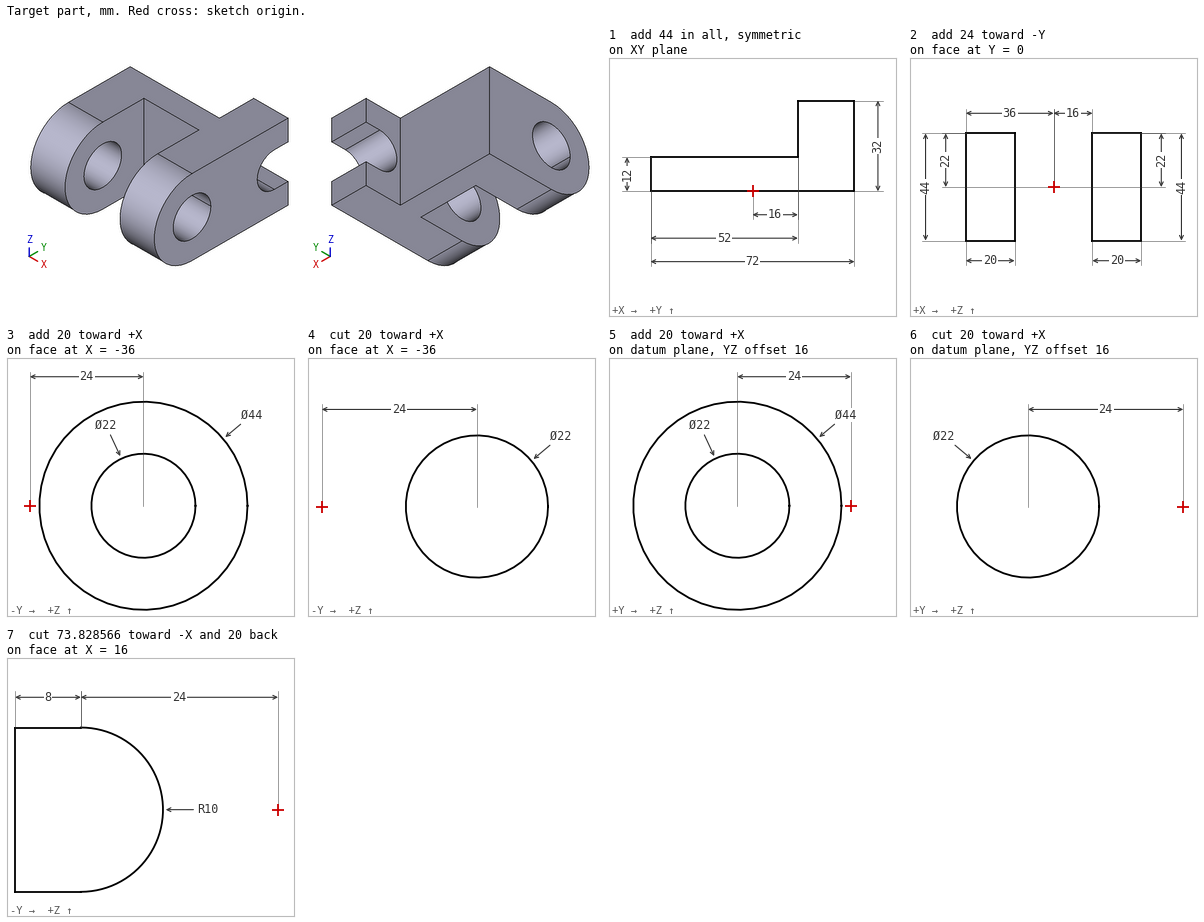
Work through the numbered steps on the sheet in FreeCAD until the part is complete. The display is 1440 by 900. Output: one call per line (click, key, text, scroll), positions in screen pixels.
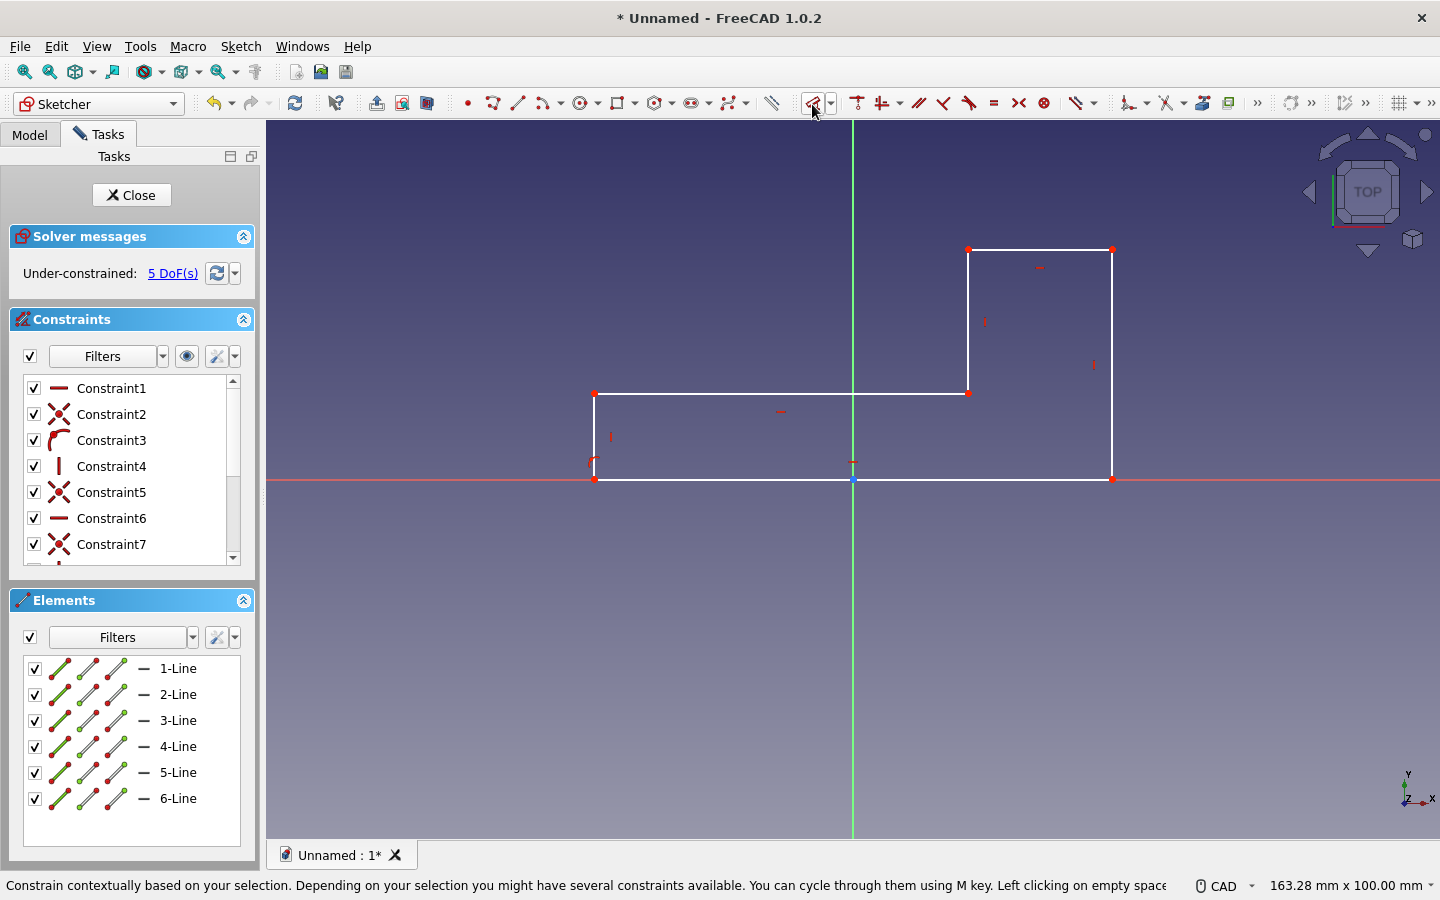
click(856, 394)
click(781, 428)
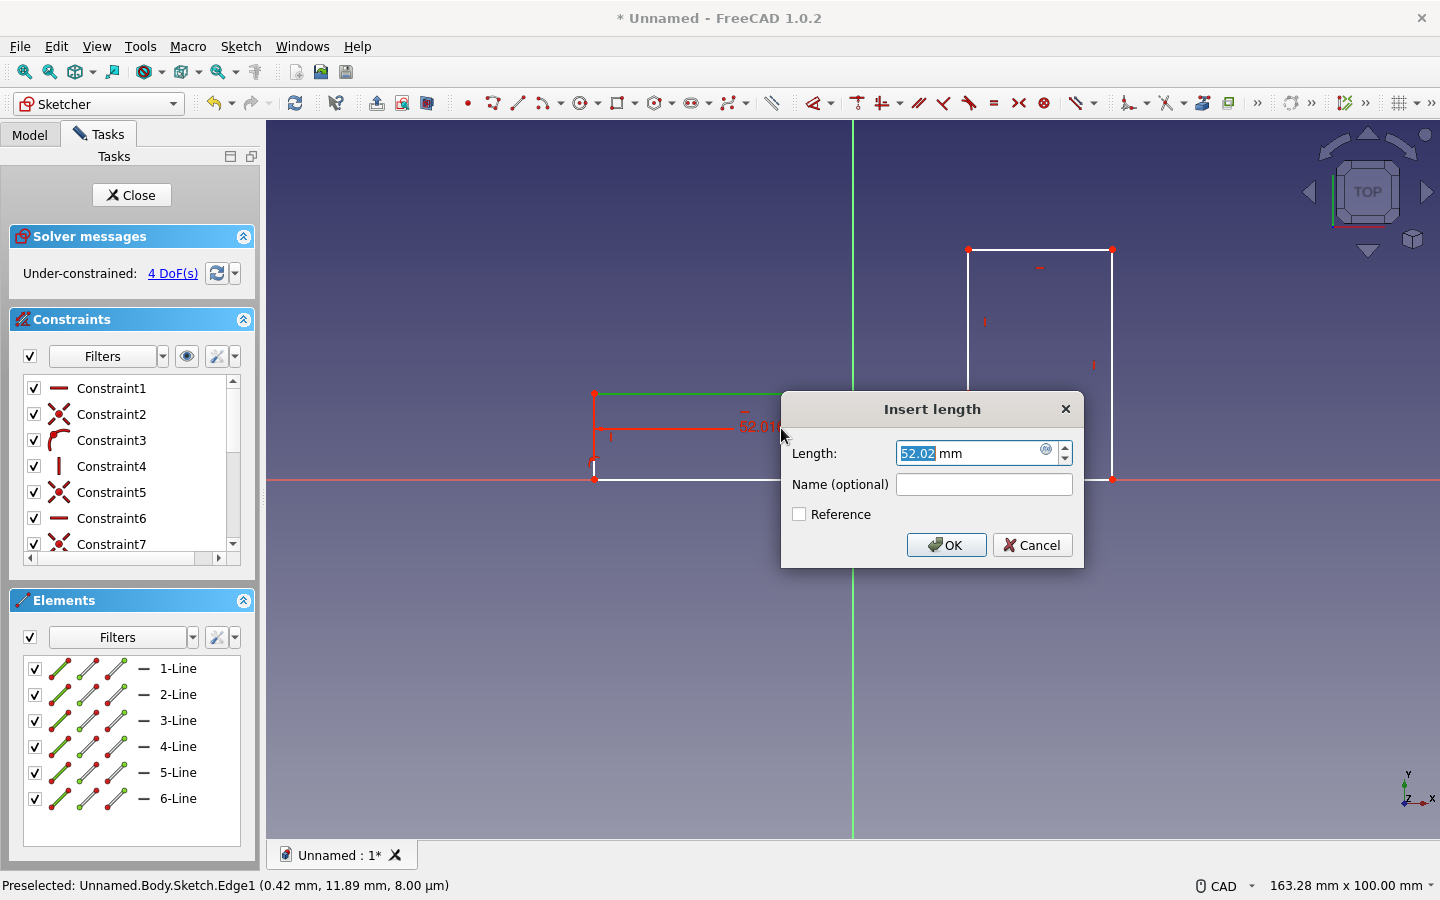
text(52)
key(Return)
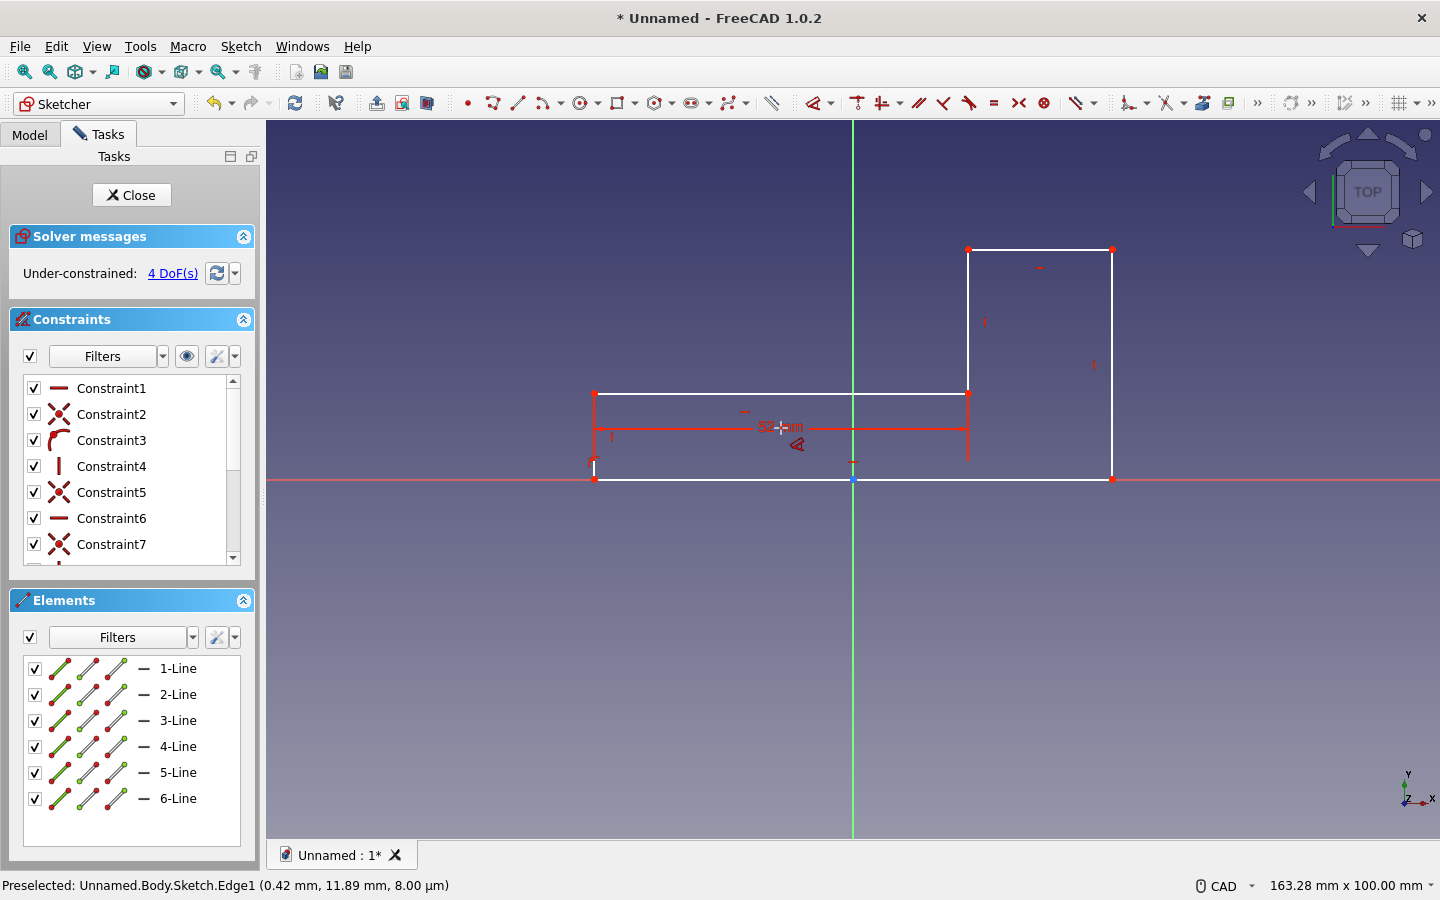
click(594, 420)
click(560, 437)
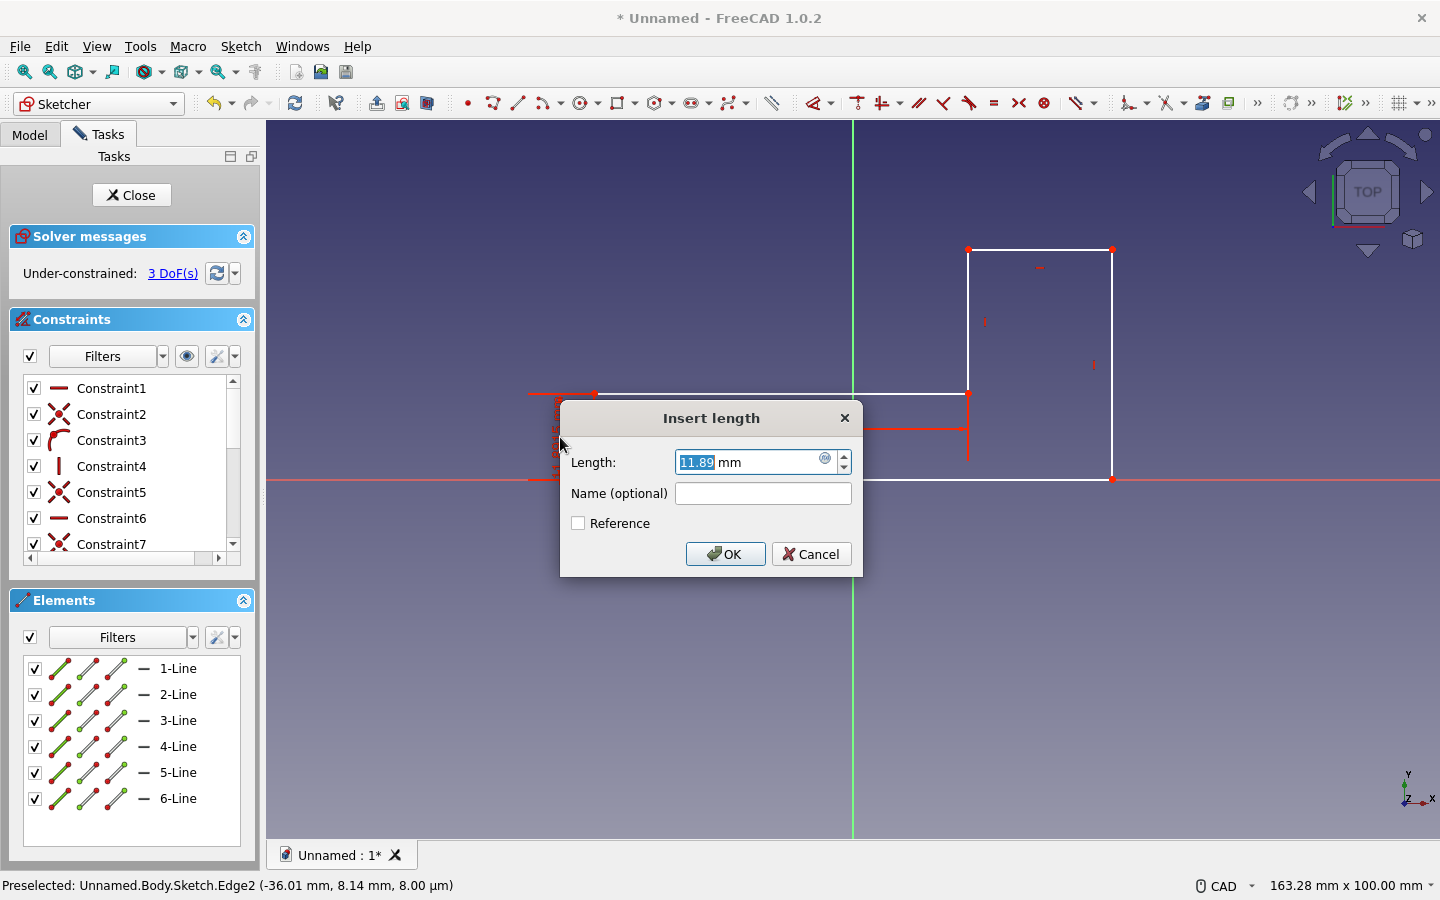
text(12)
key(Return)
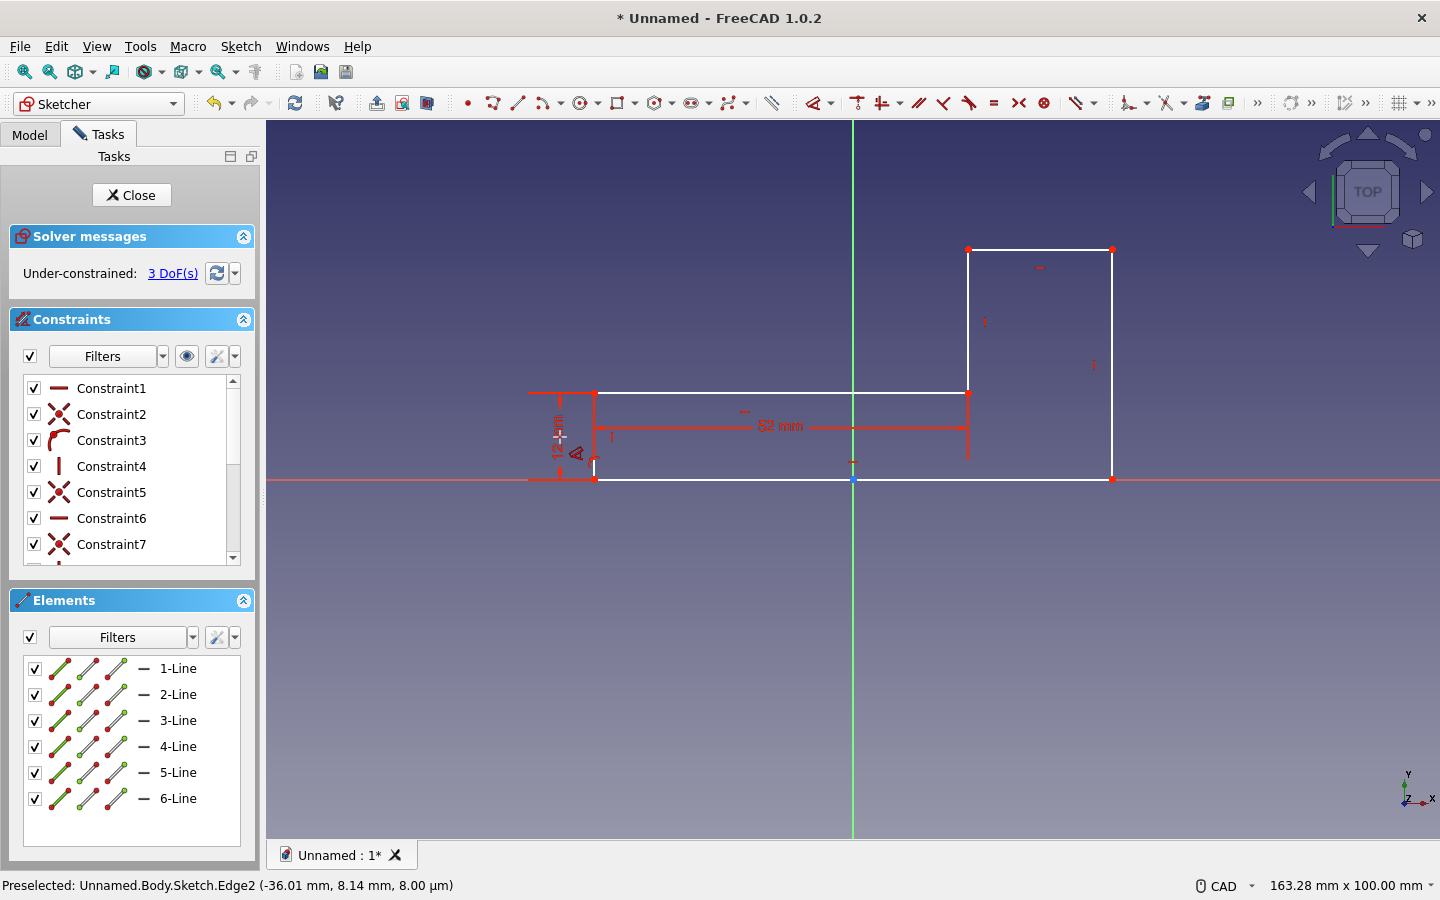
click(749, 480)
click(734, 514)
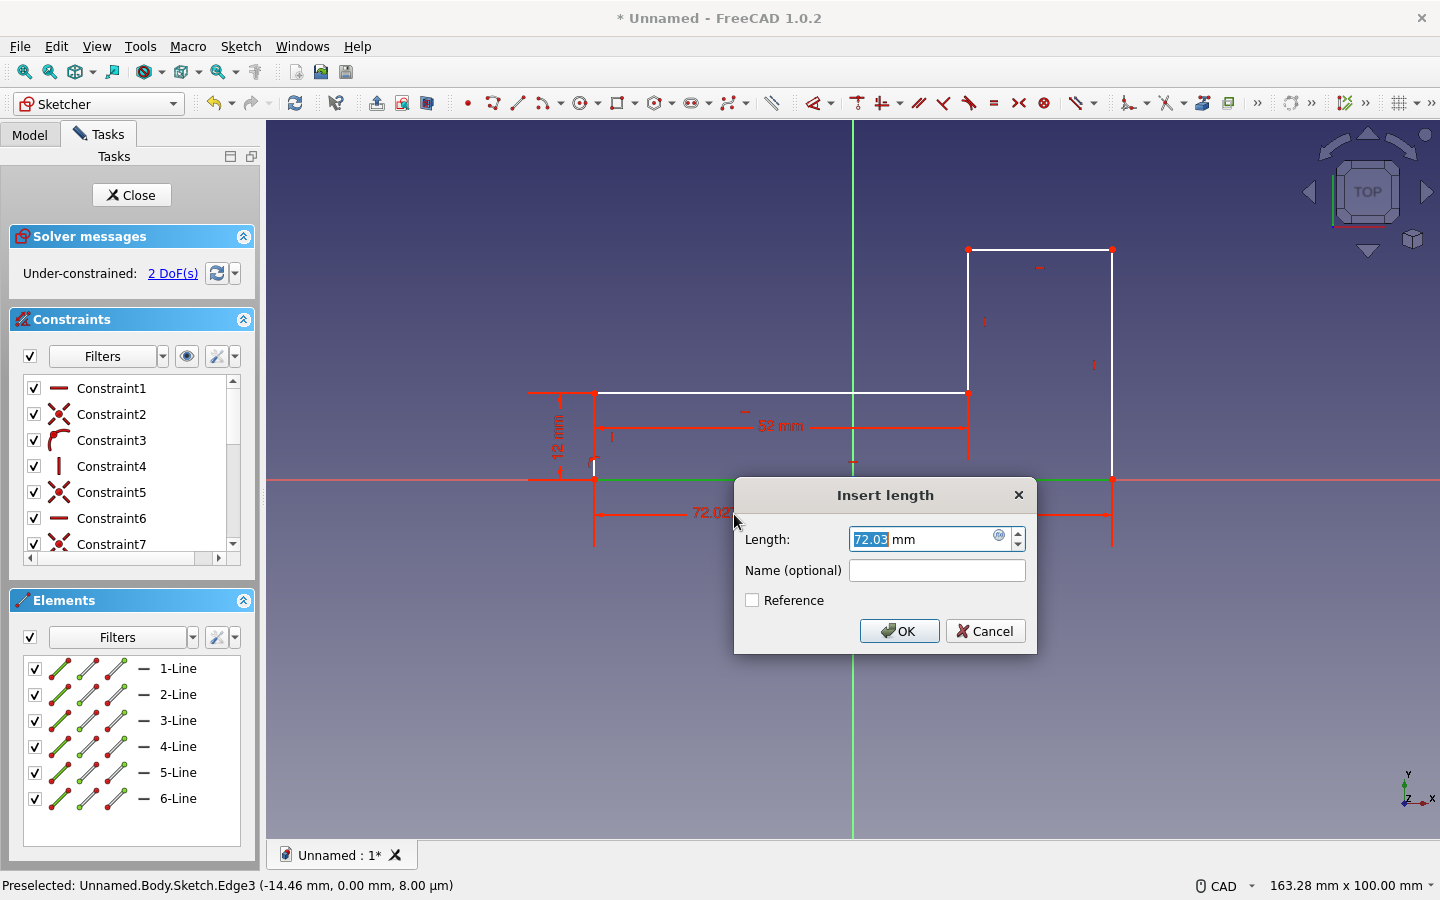
text(72)
key(Return)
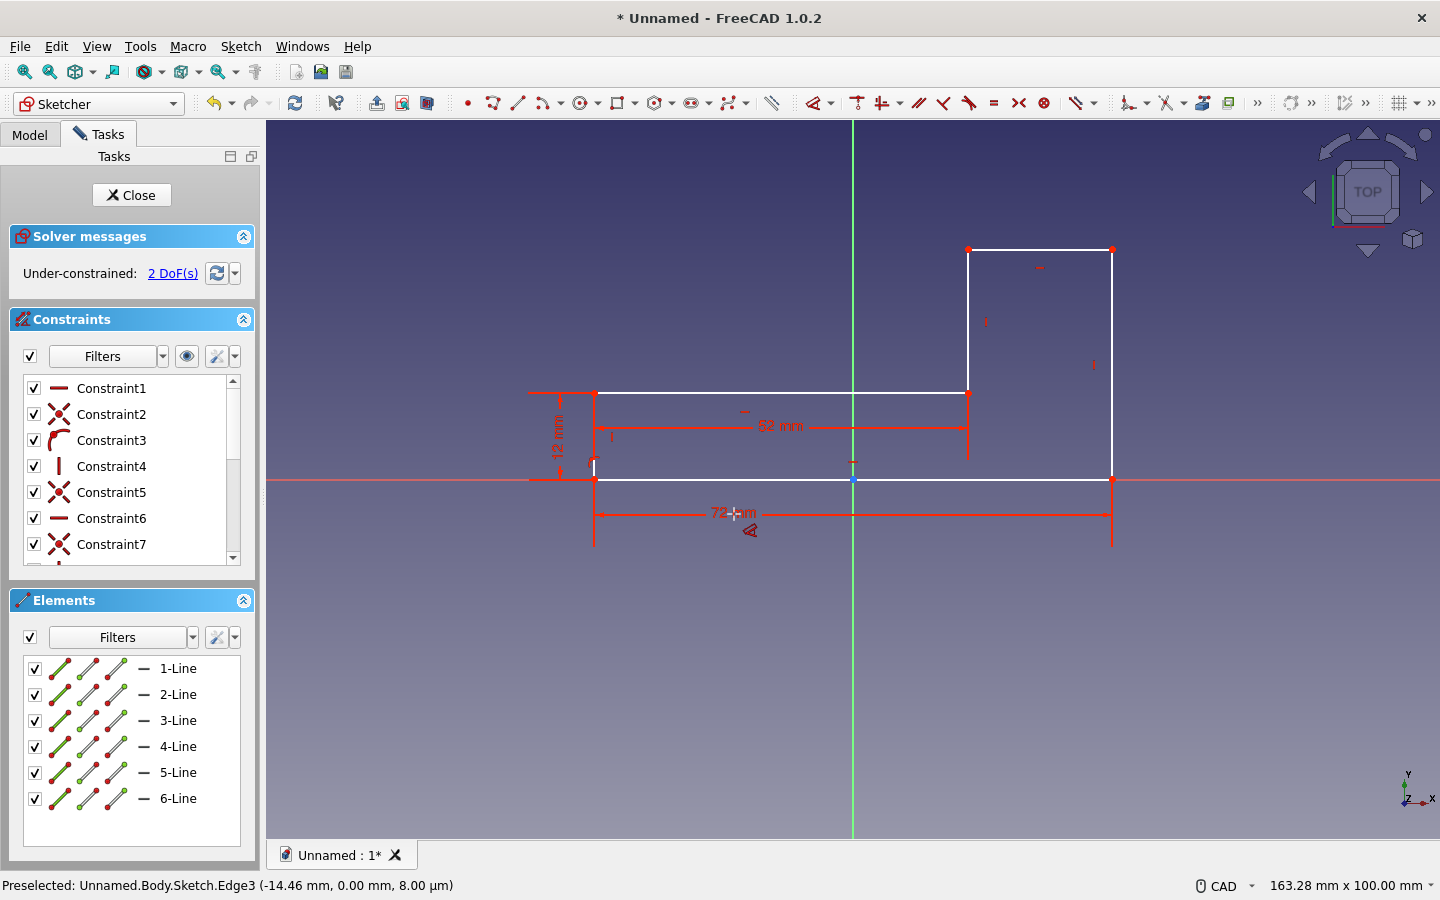
click(1112, 411)
click(1146, 365)